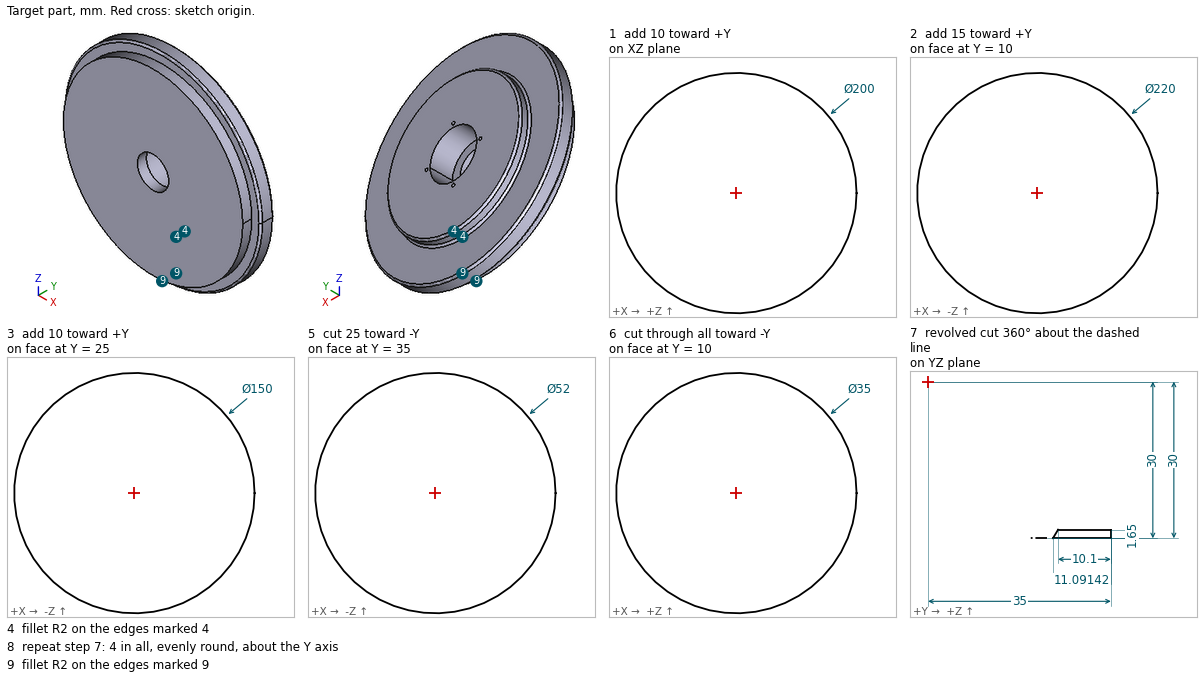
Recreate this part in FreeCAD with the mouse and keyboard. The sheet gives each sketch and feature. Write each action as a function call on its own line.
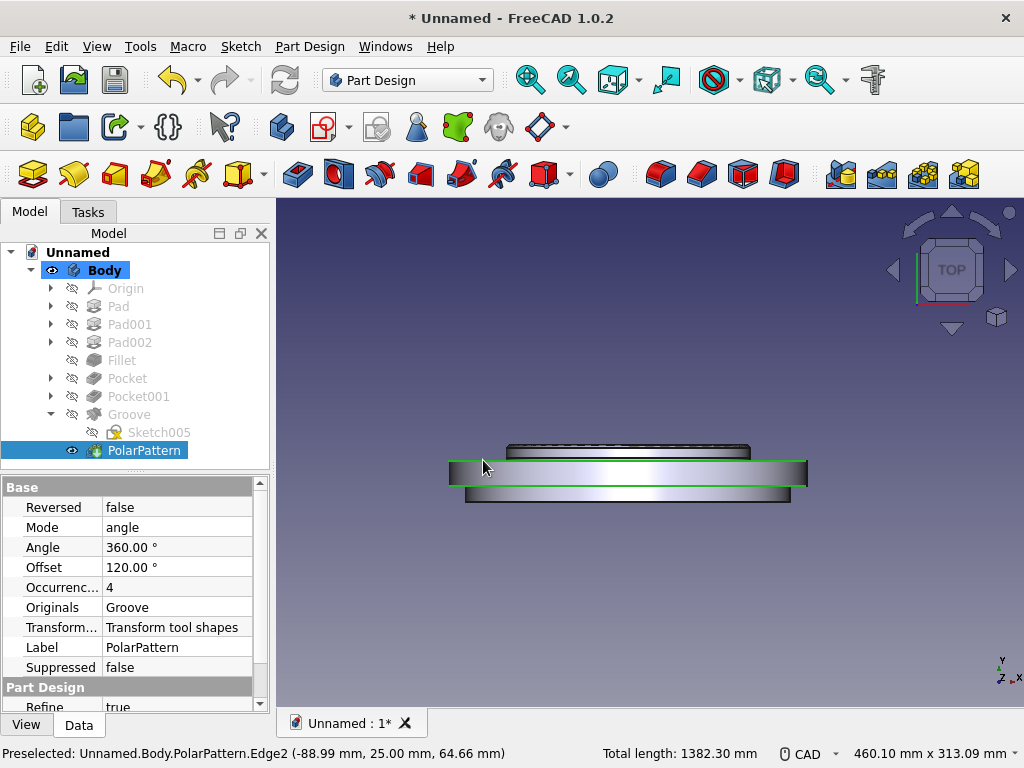
click(661, 174)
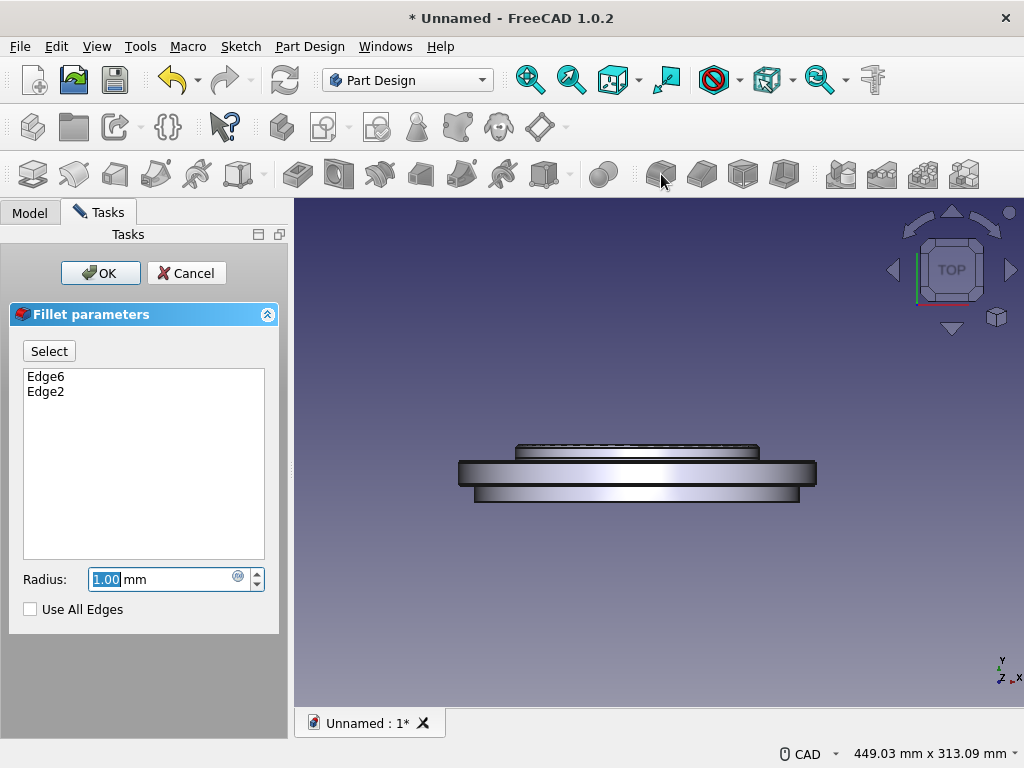
text(2)
key(Tab)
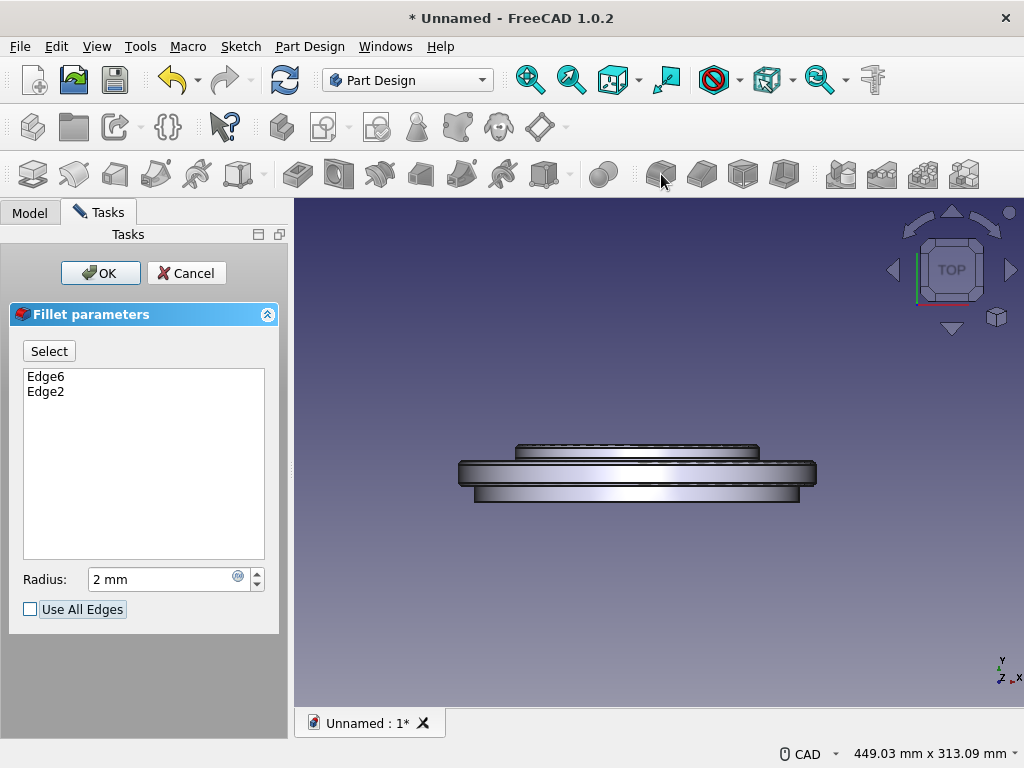
click(101, 273)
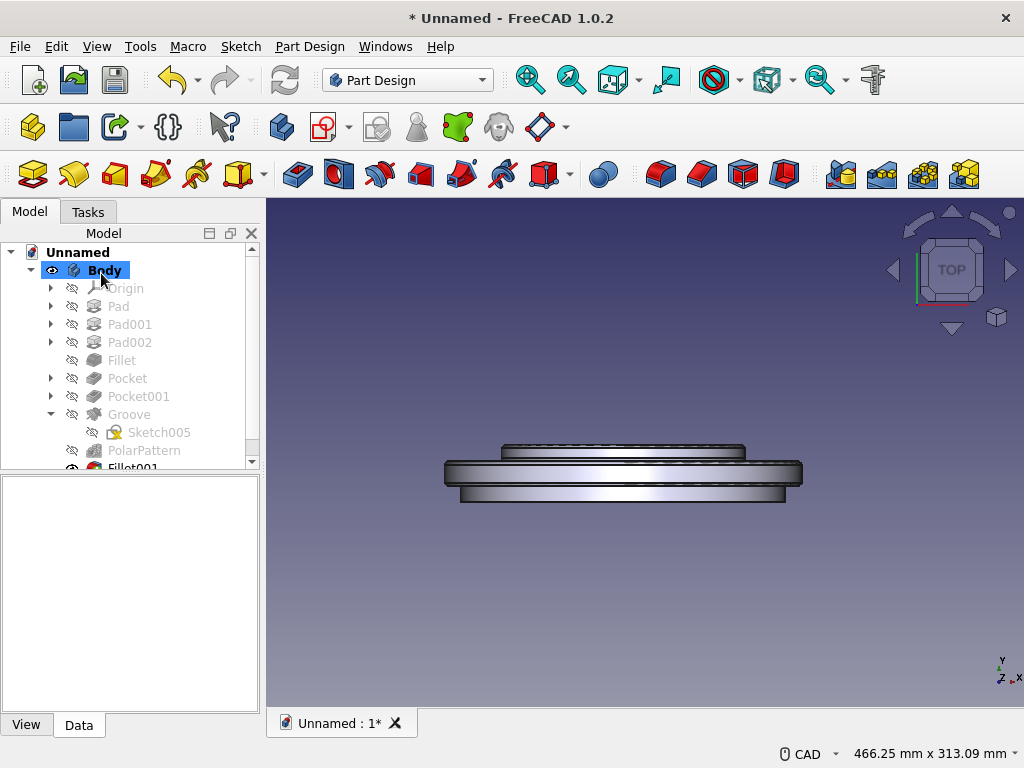
key(0)